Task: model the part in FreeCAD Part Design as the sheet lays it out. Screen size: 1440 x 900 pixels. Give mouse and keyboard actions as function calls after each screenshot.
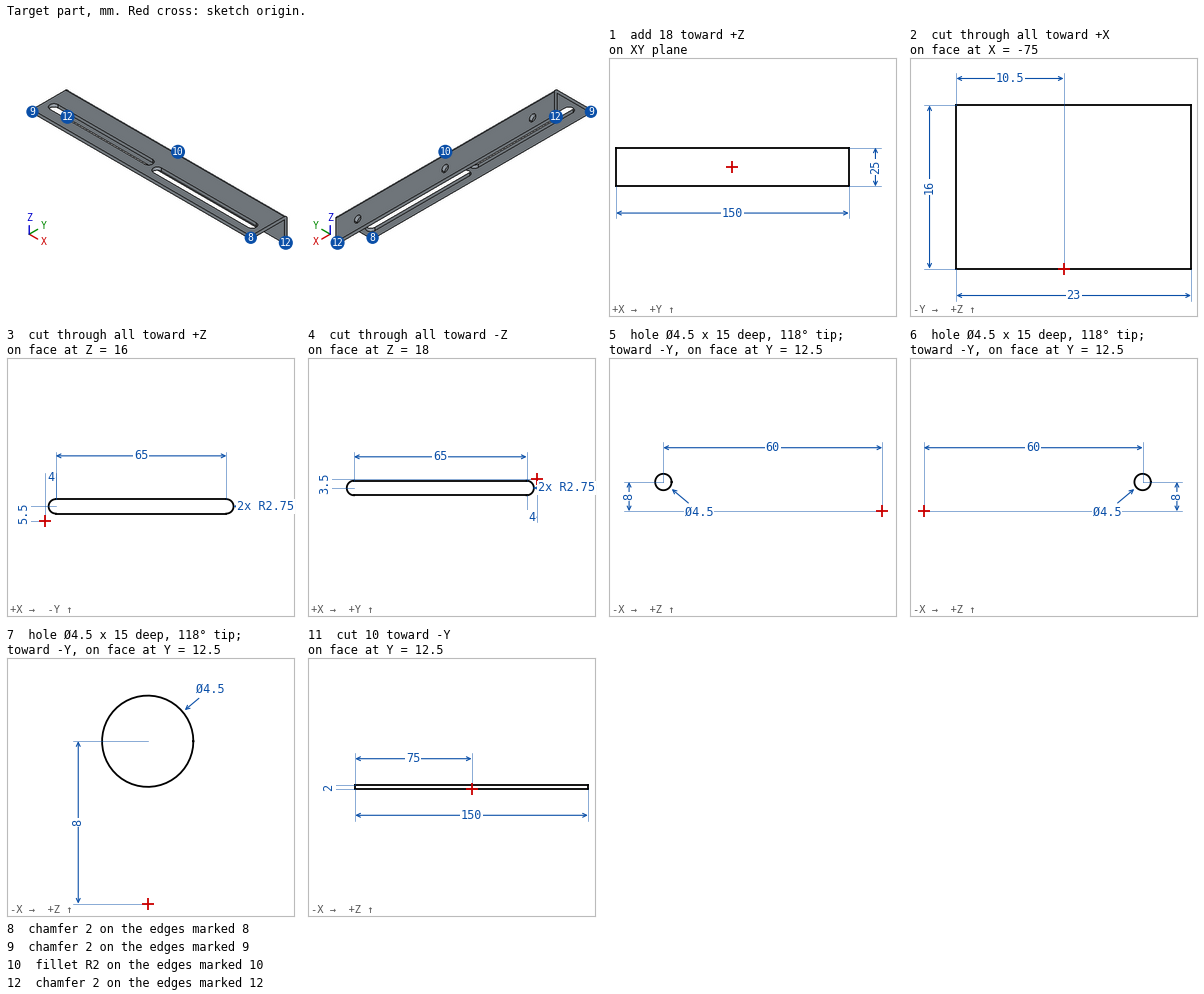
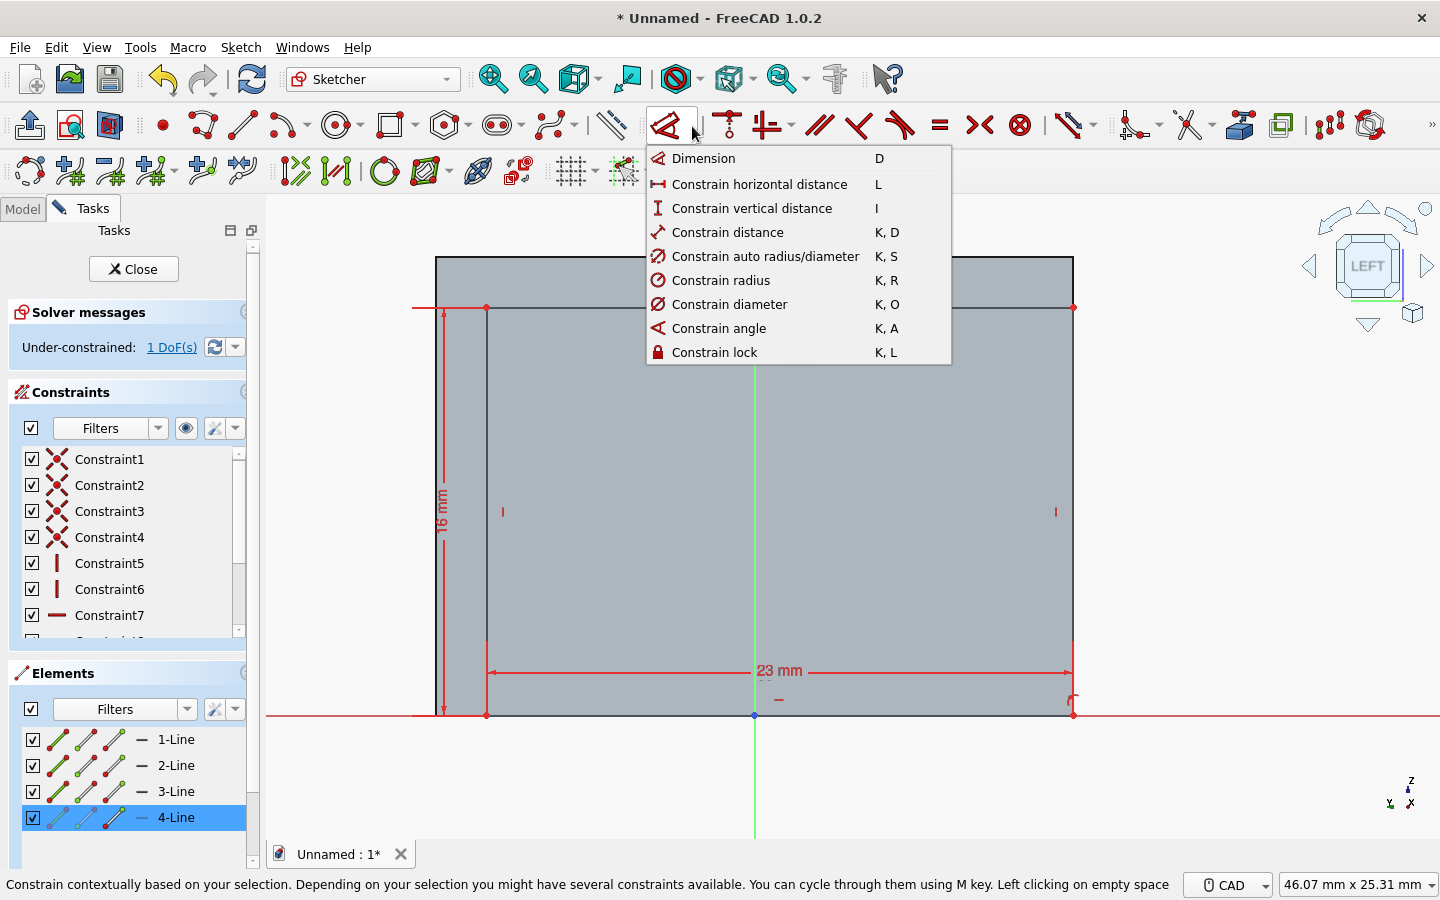
click(799, 184)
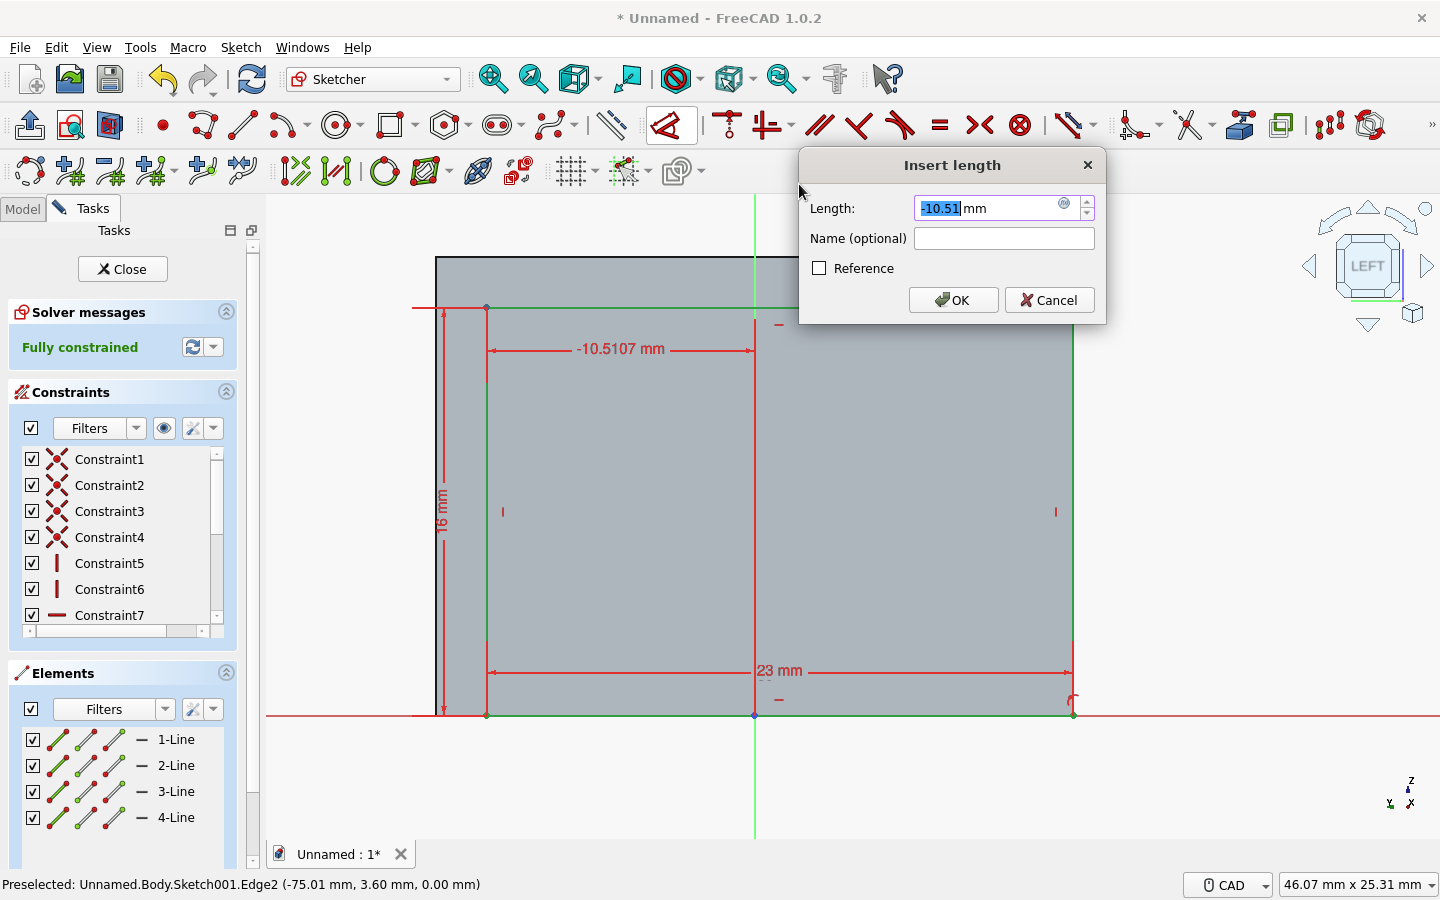
text(-10.5)
key(Return)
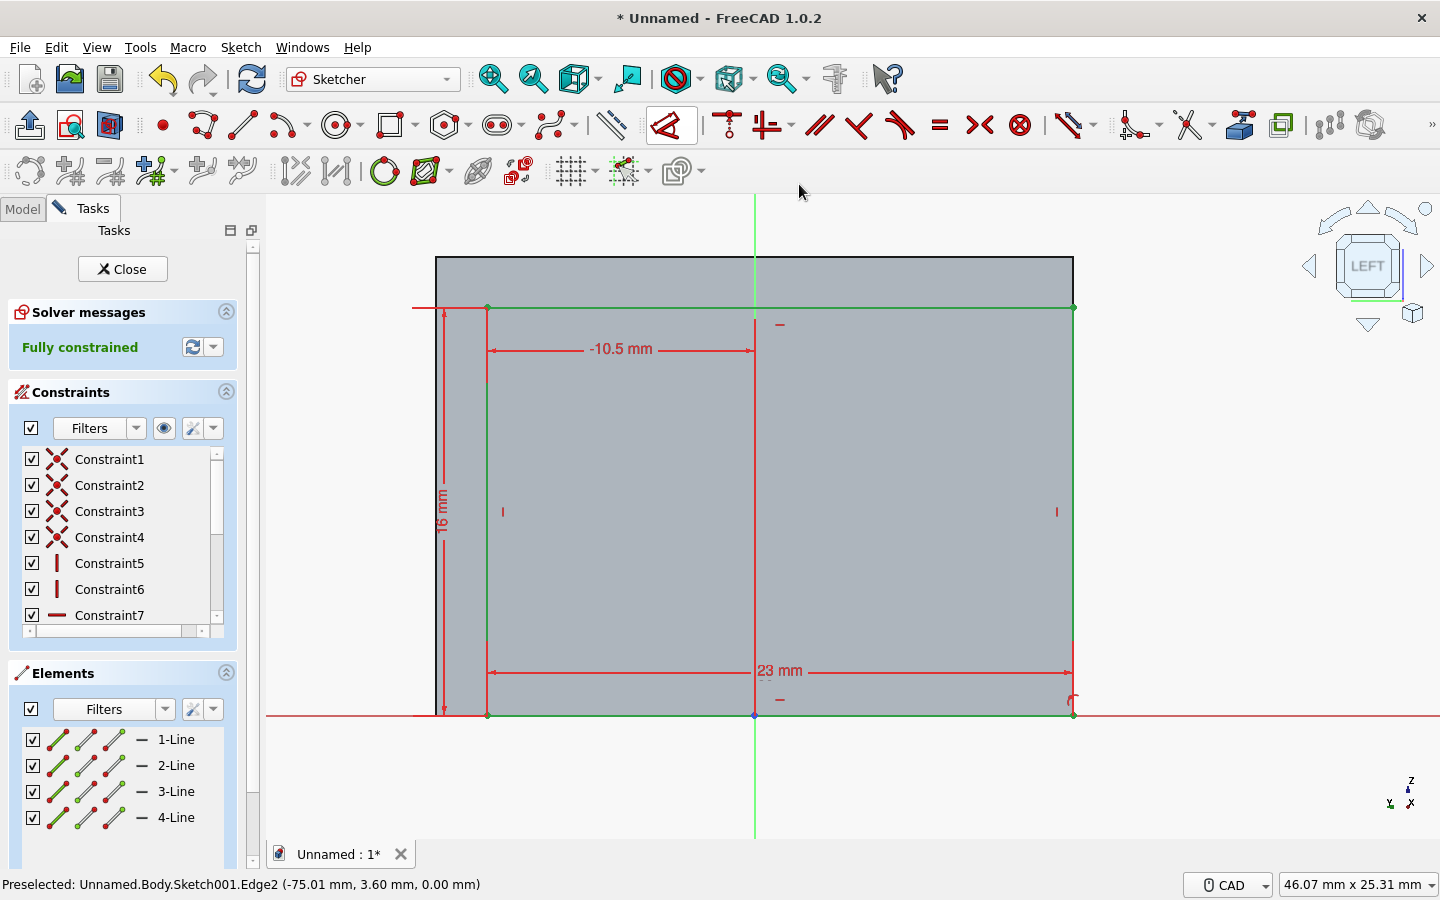
click(123, 269)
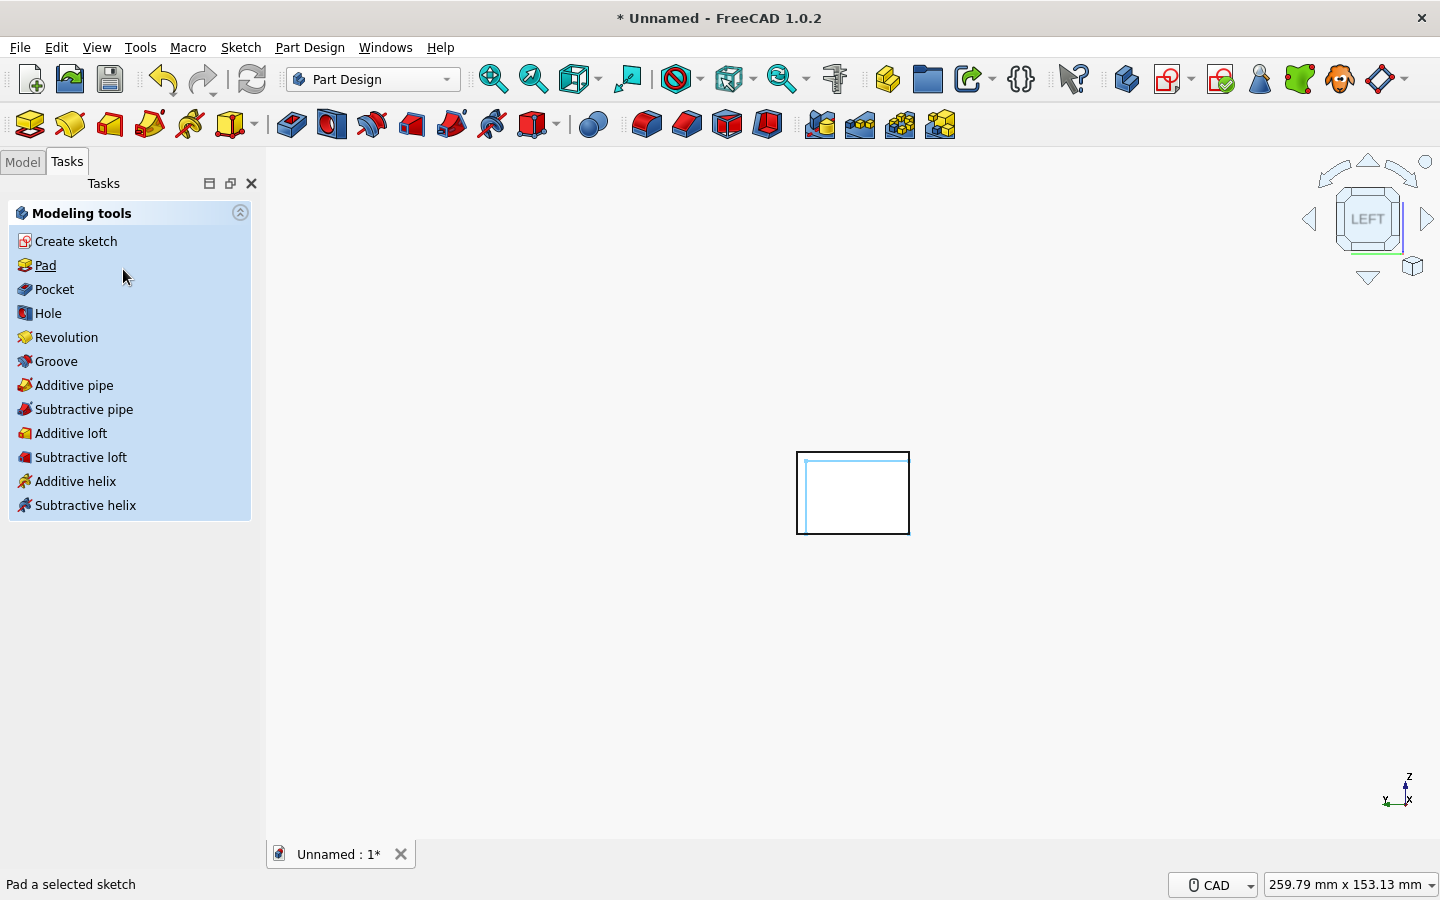
click(292, 124)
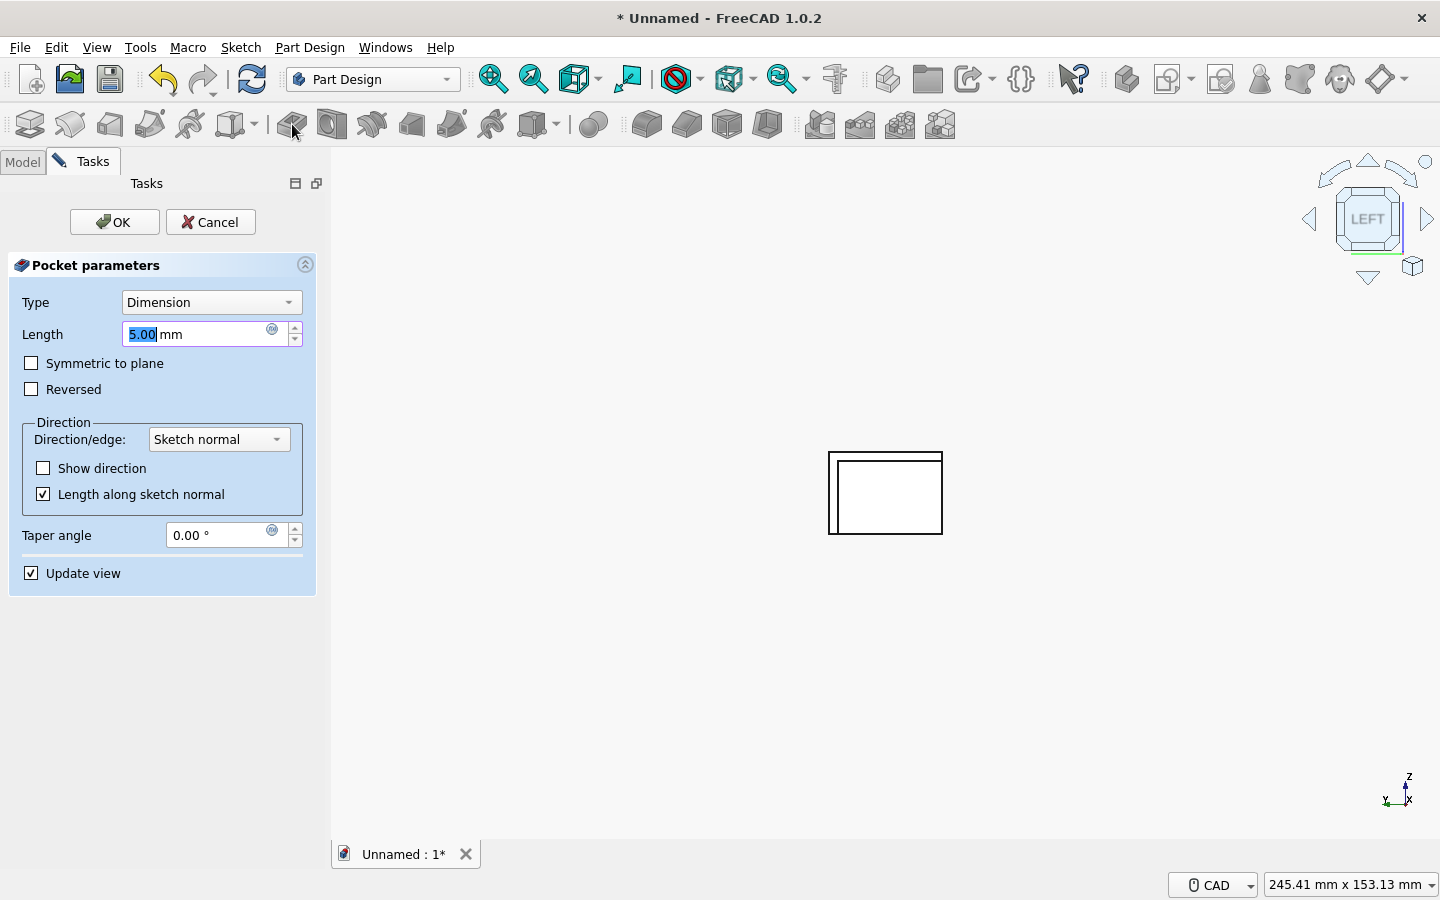
click(212, 302)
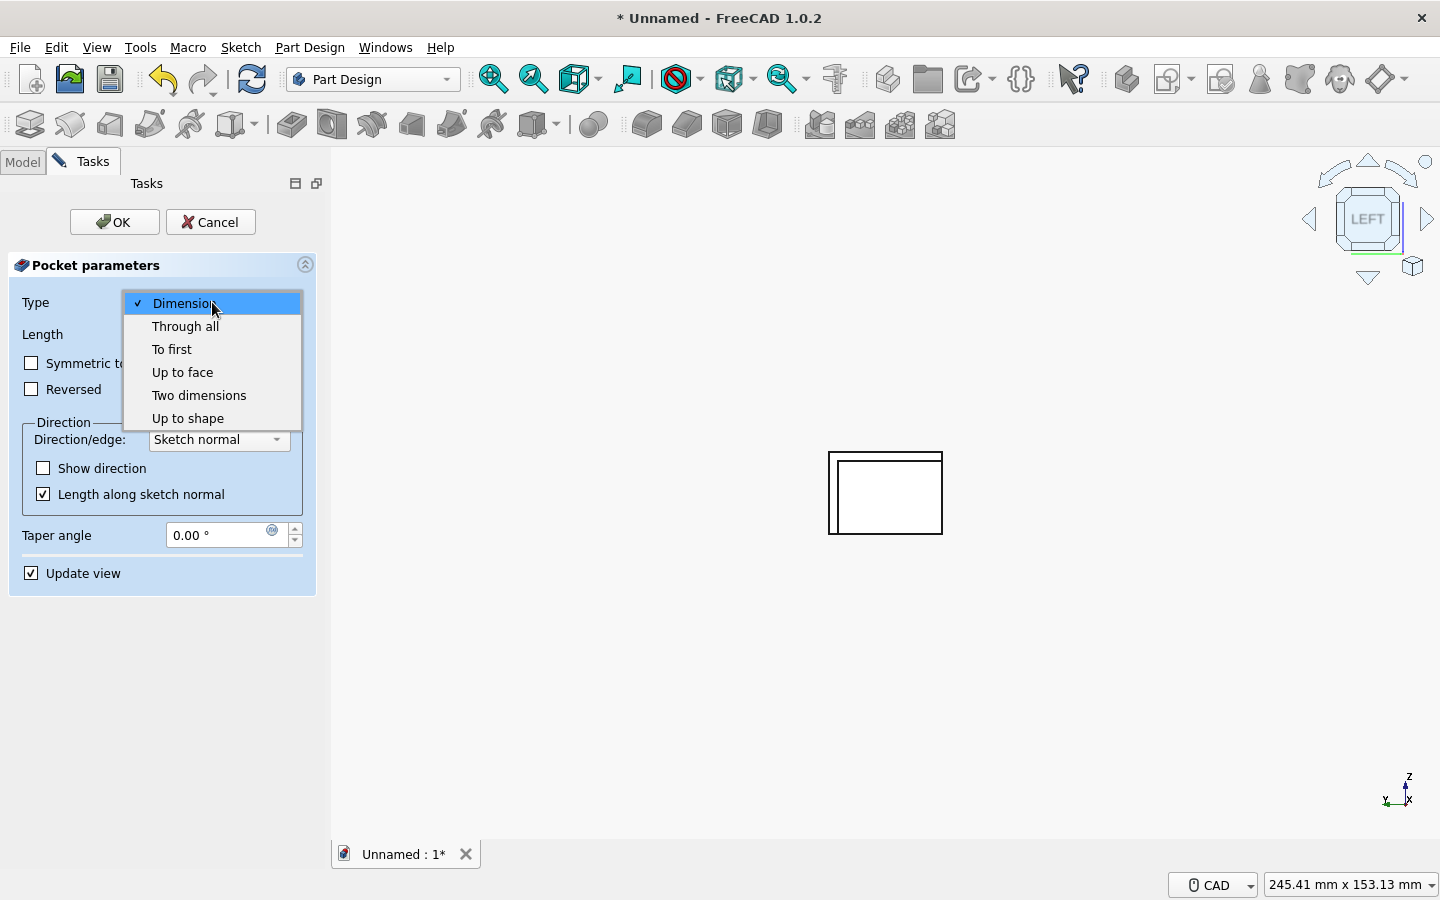
click(212, 326)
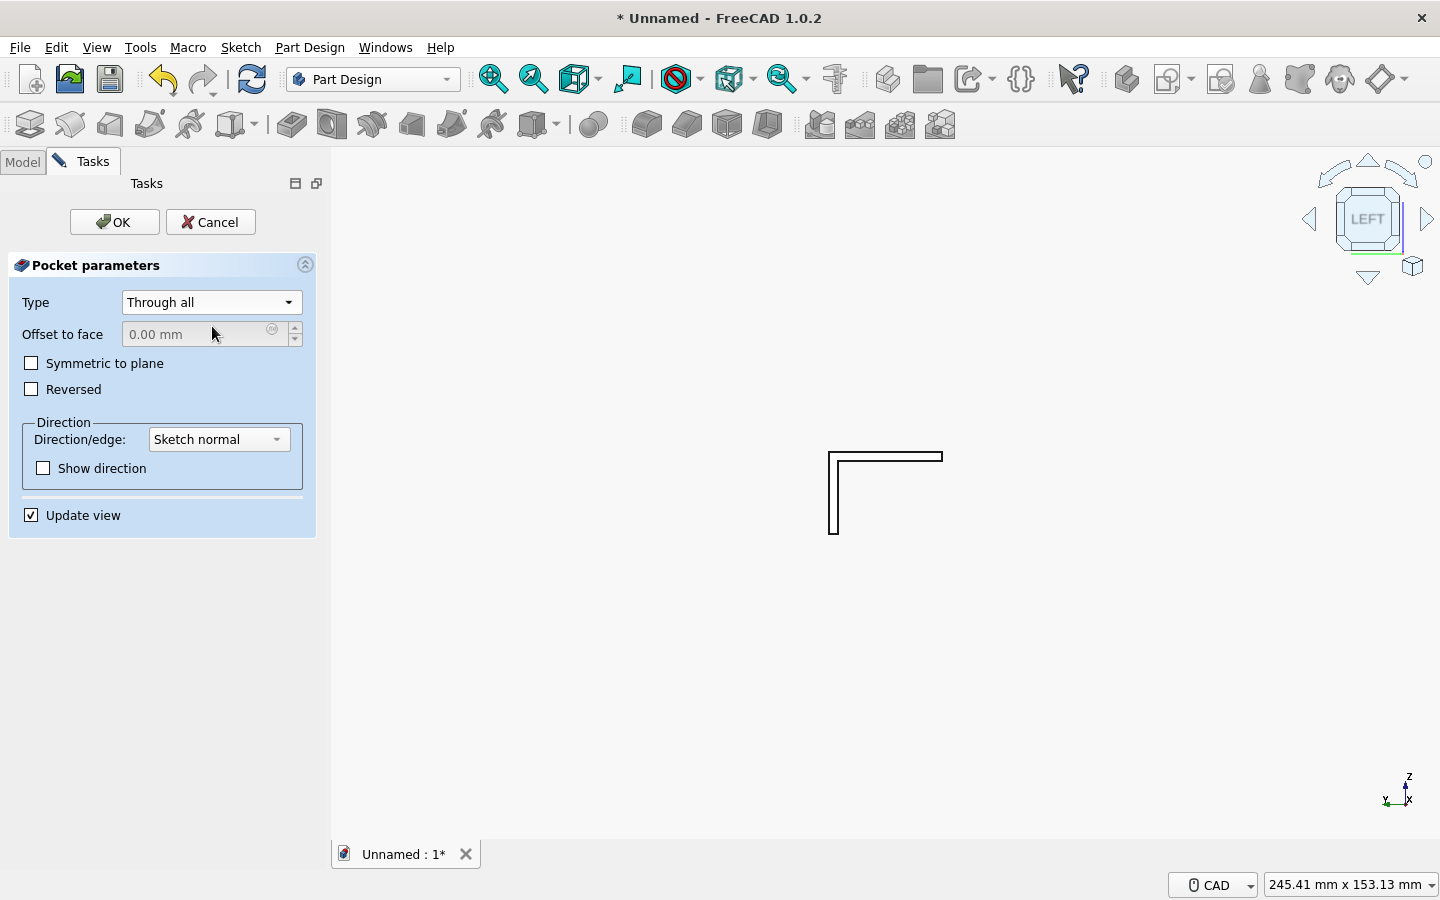
click(115, 222)